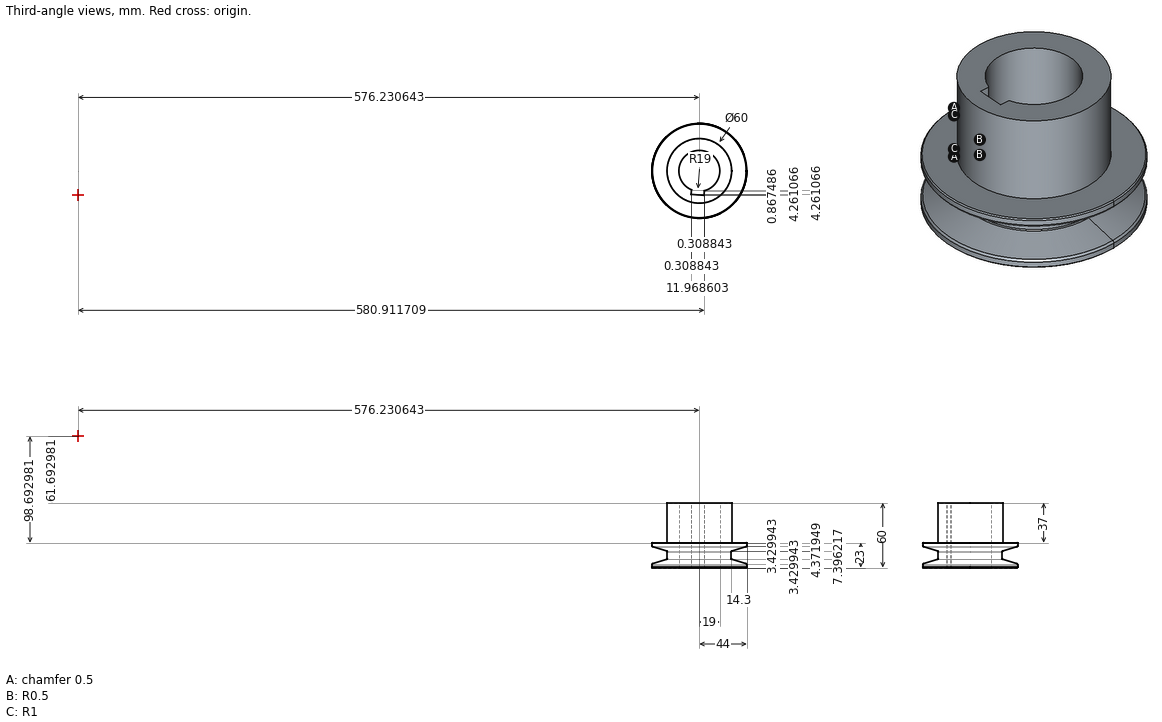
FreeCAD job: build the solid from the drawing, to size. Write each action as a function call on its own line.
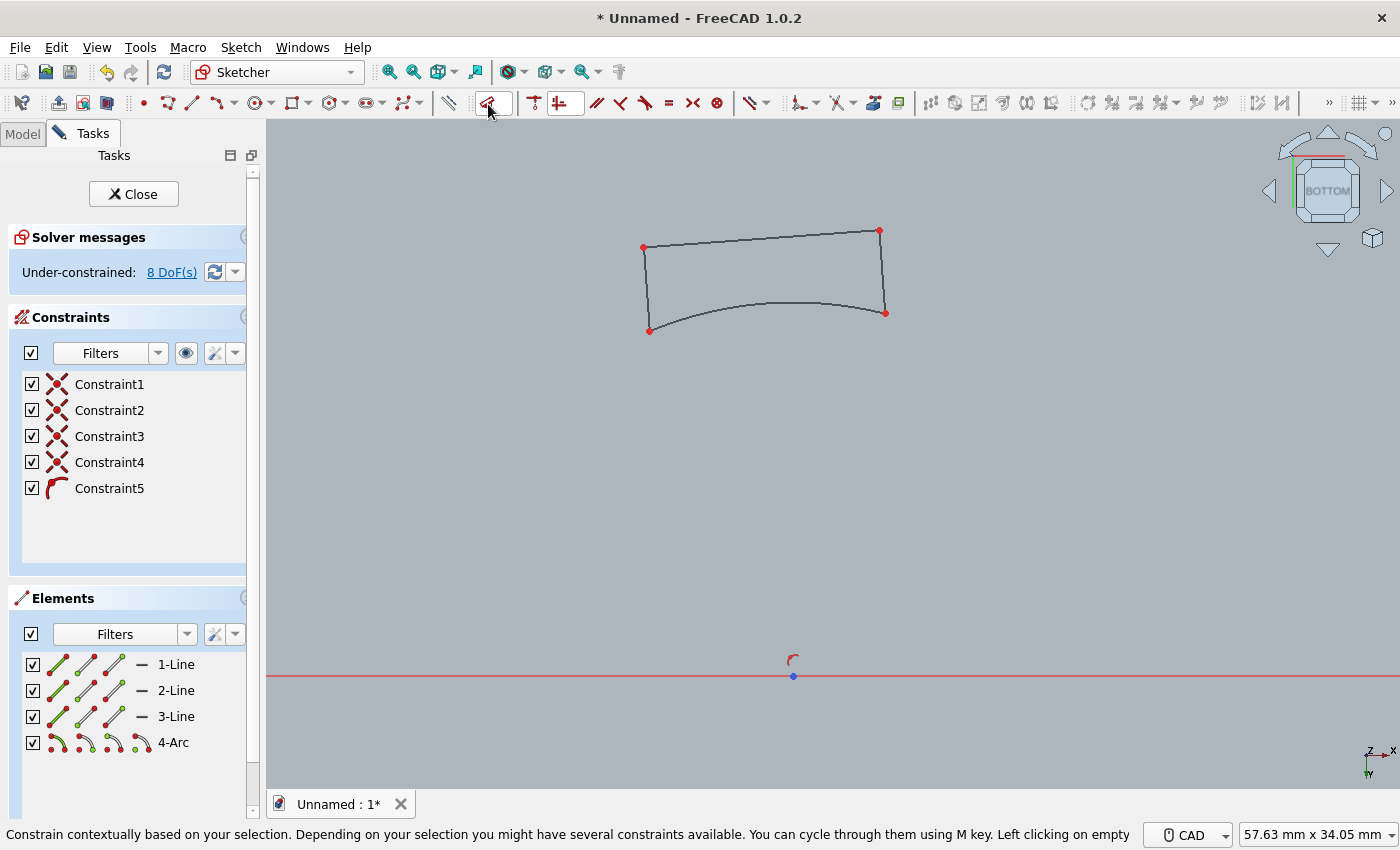
click(814, 303)
click(816, 271)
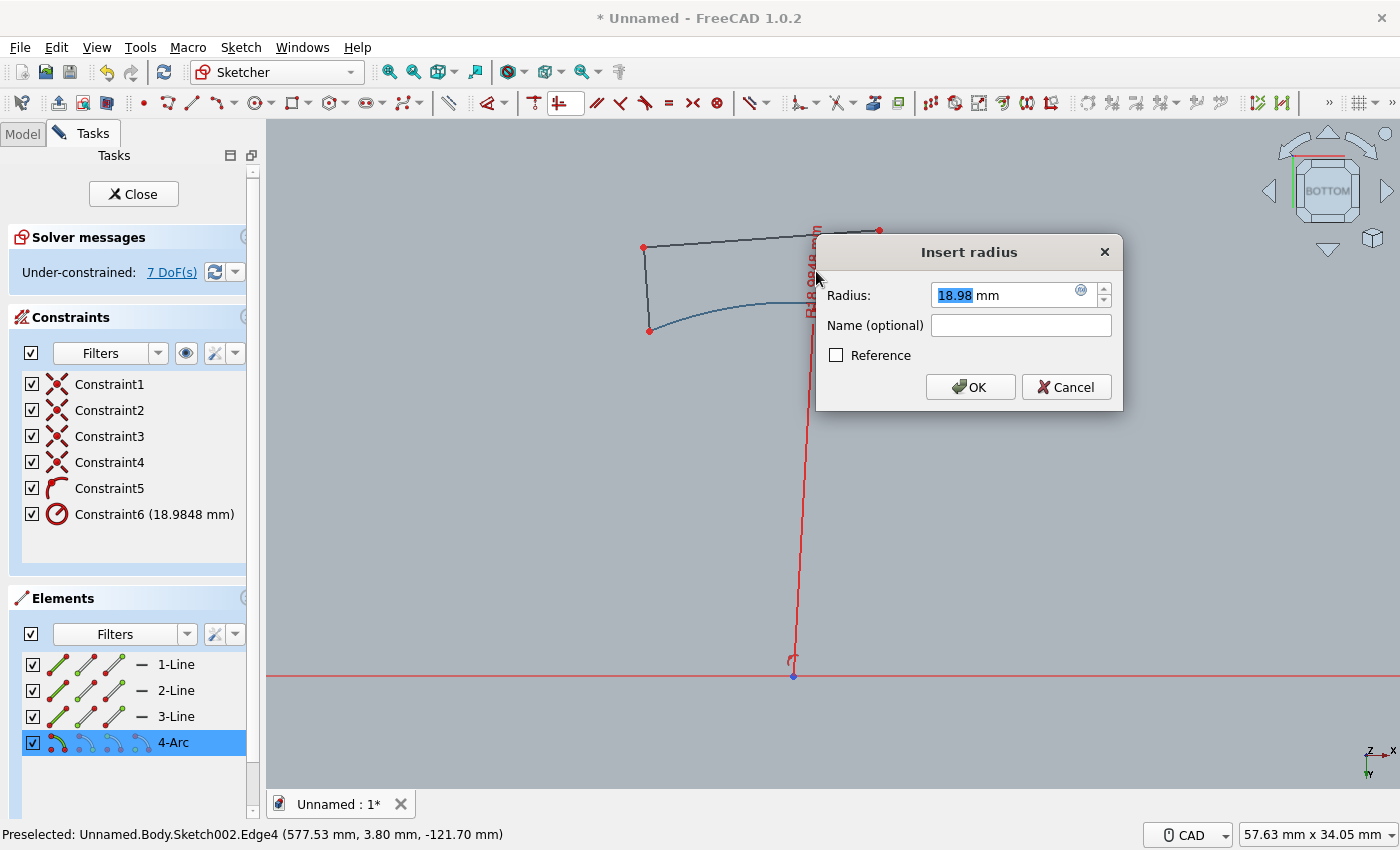
text(19)
key(Return)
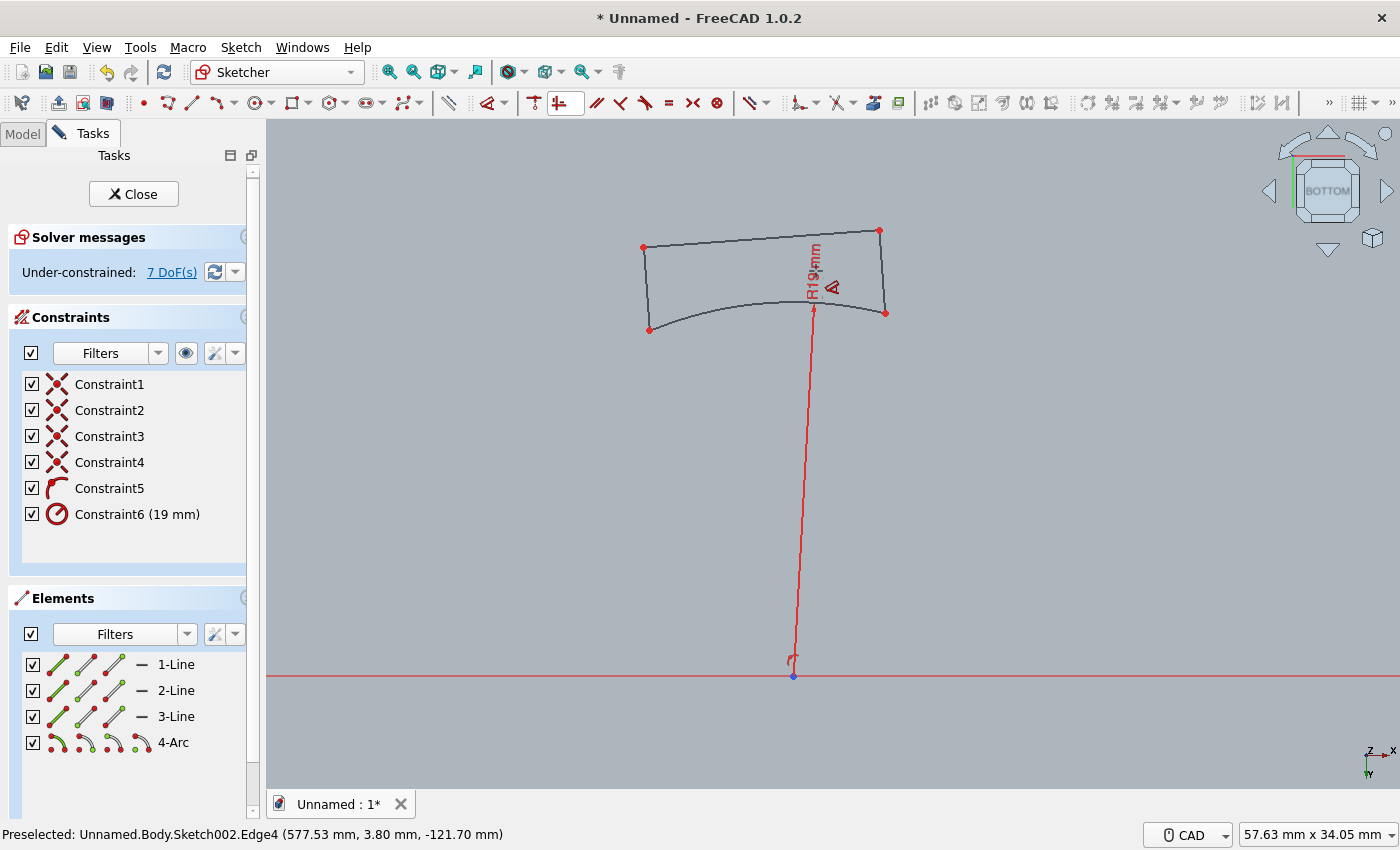
scroll(884, 289, up, 10)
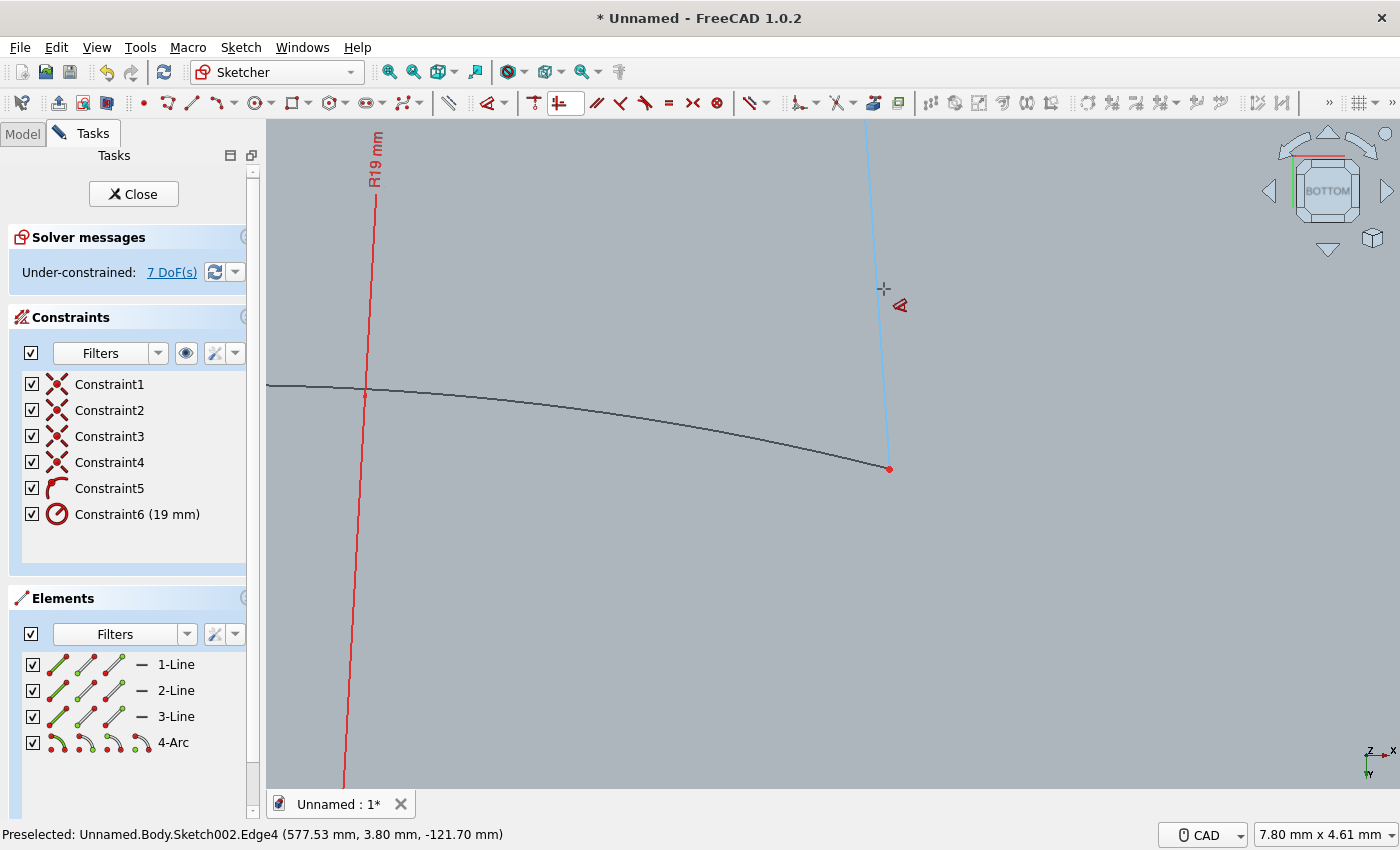
click(877, 284)
click(868, 503)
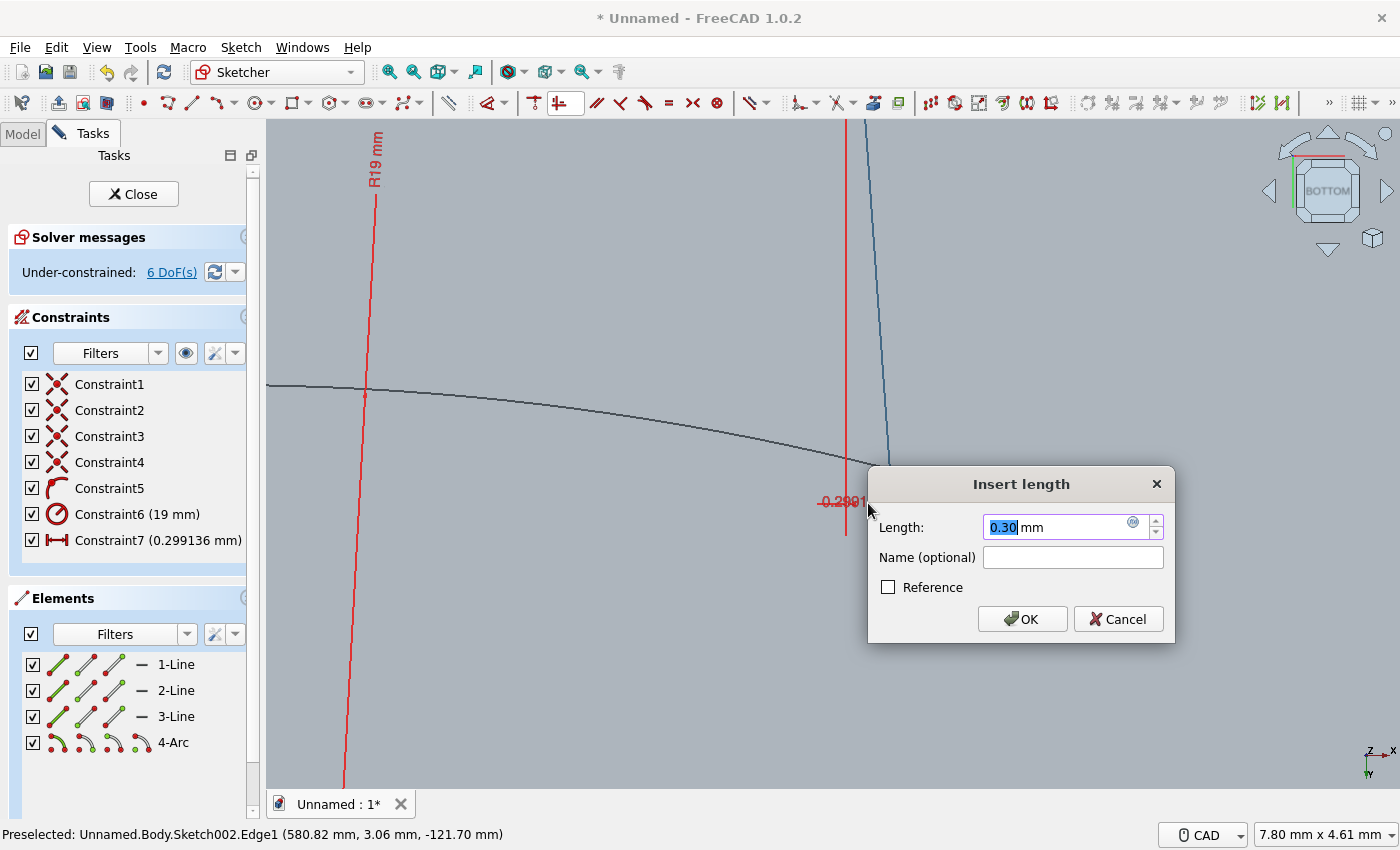
text(0.308843)
key(Return)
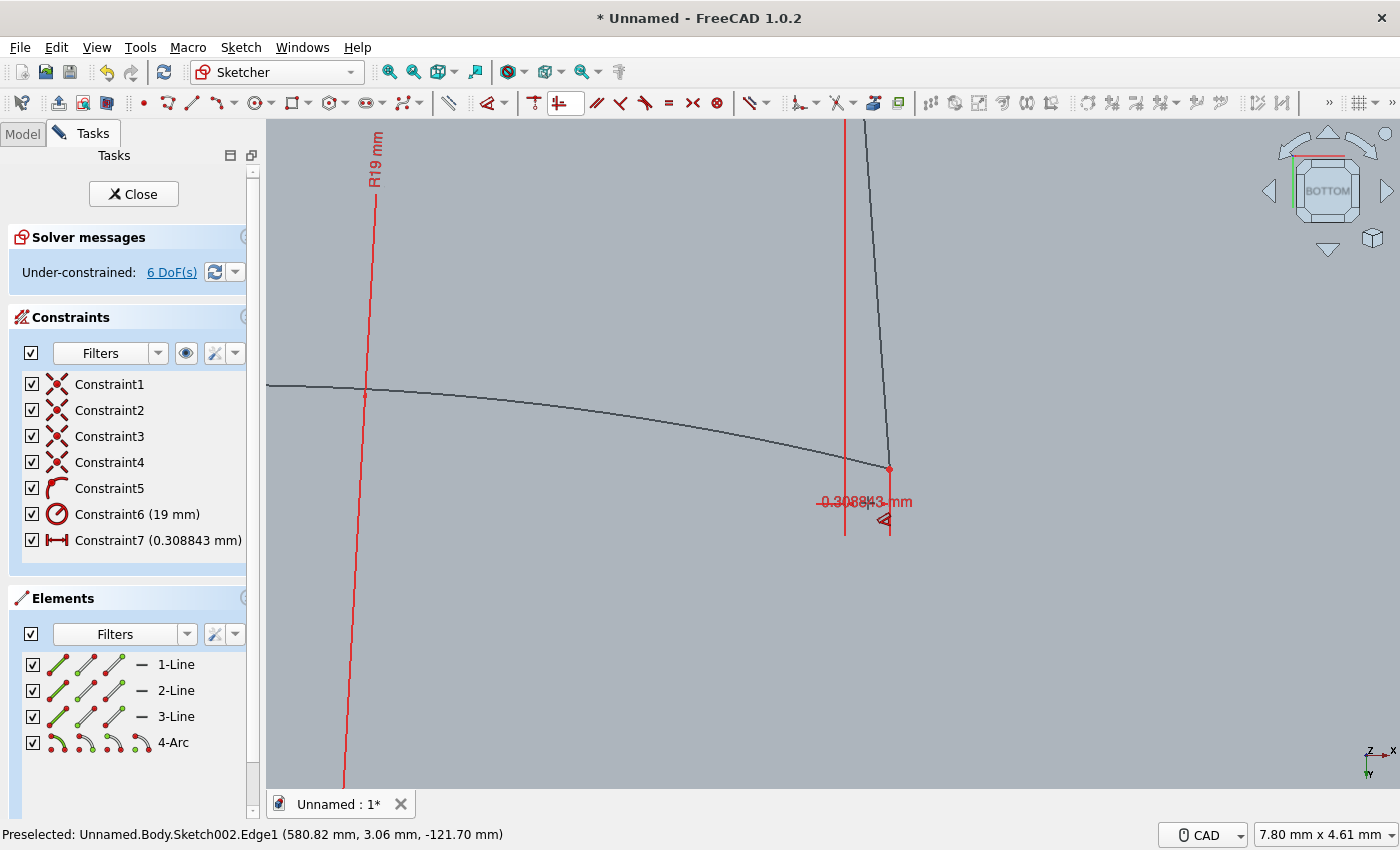
click(876, 284)
click(924, 308)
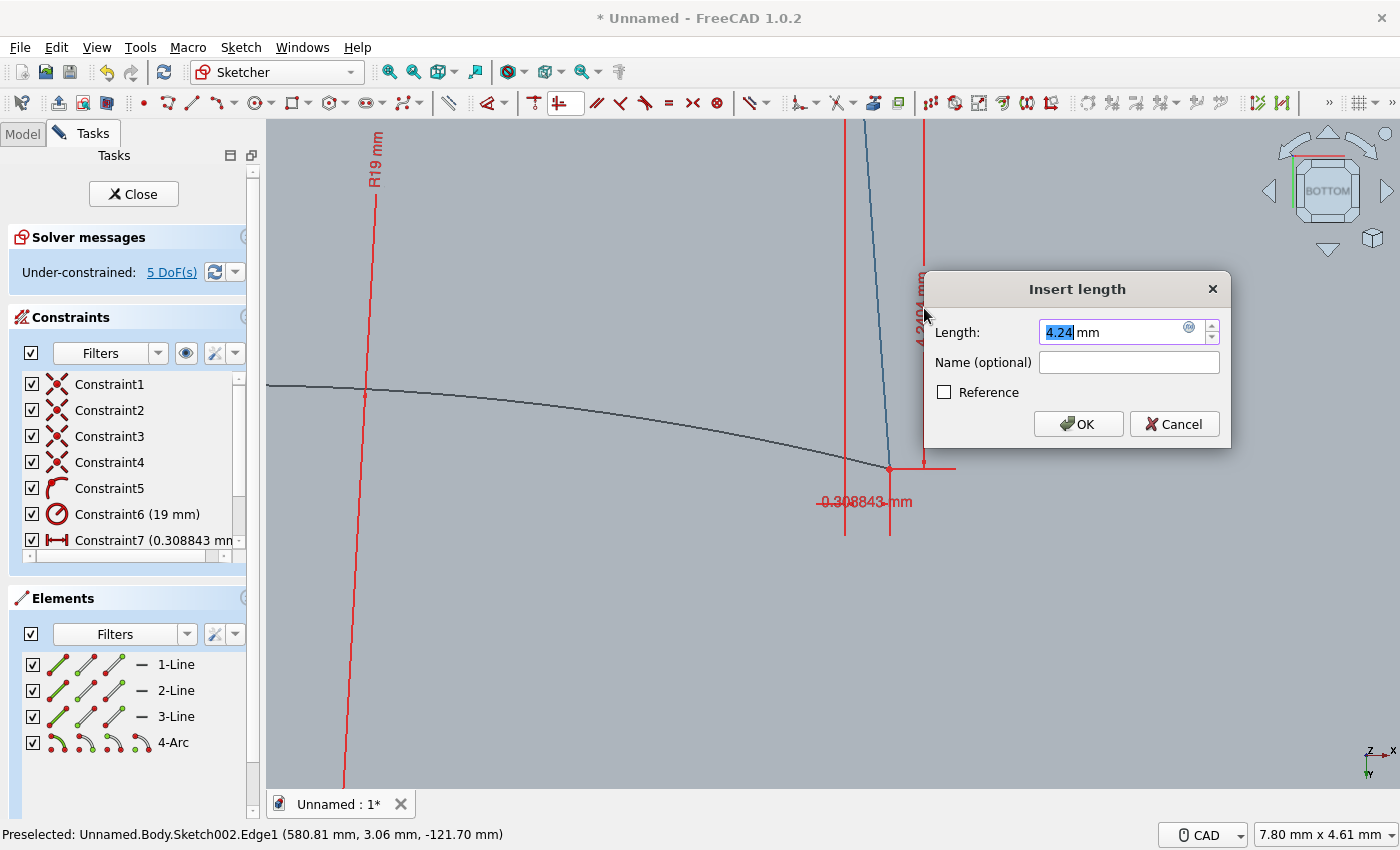
text(4.261066)
key(Return)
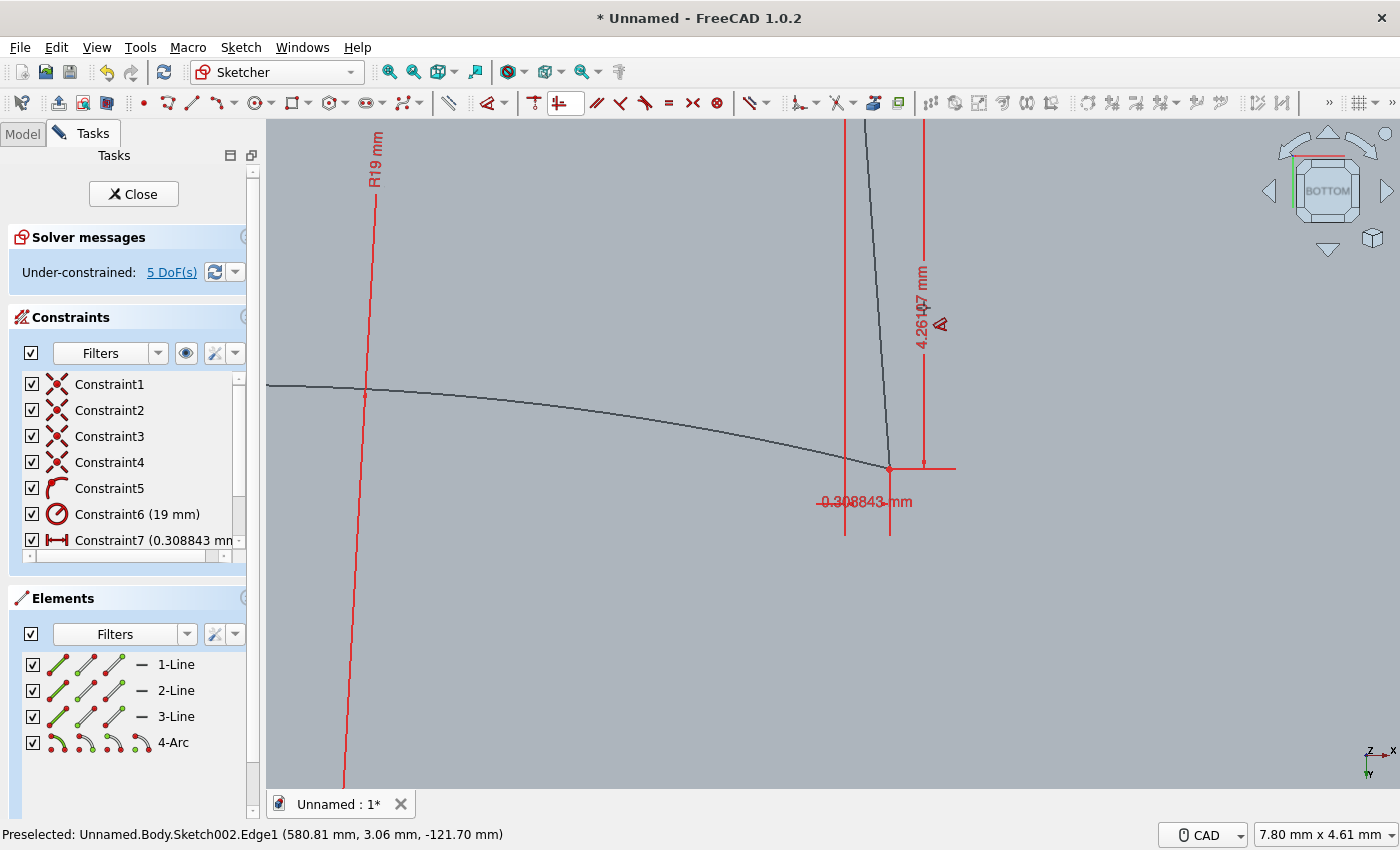
scroll(1210, 588, down, 5)